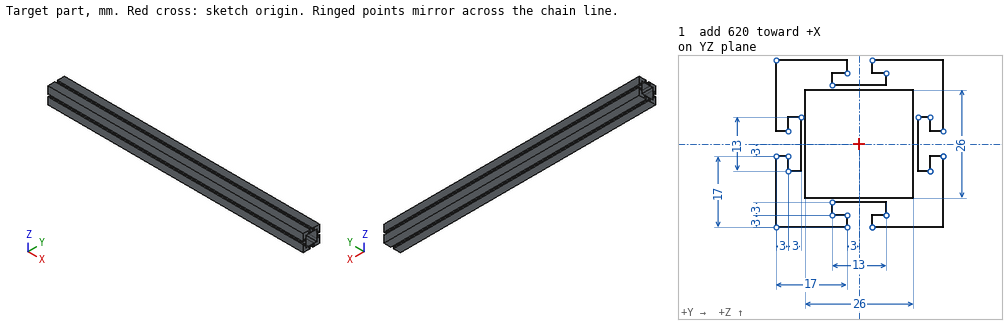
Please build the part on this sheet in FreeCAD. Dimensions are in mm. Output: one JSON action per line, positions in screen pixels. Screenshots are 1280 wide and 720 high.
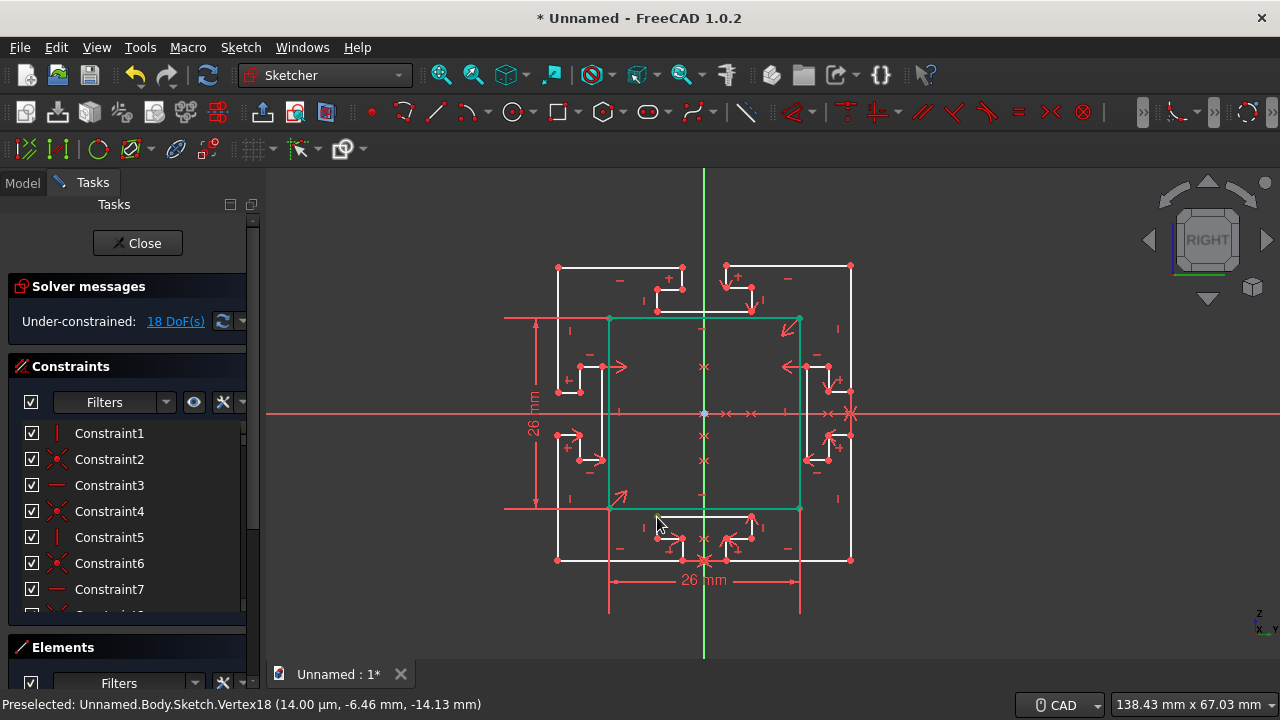
{"action": "left_click", "coordinate": [657, 312]}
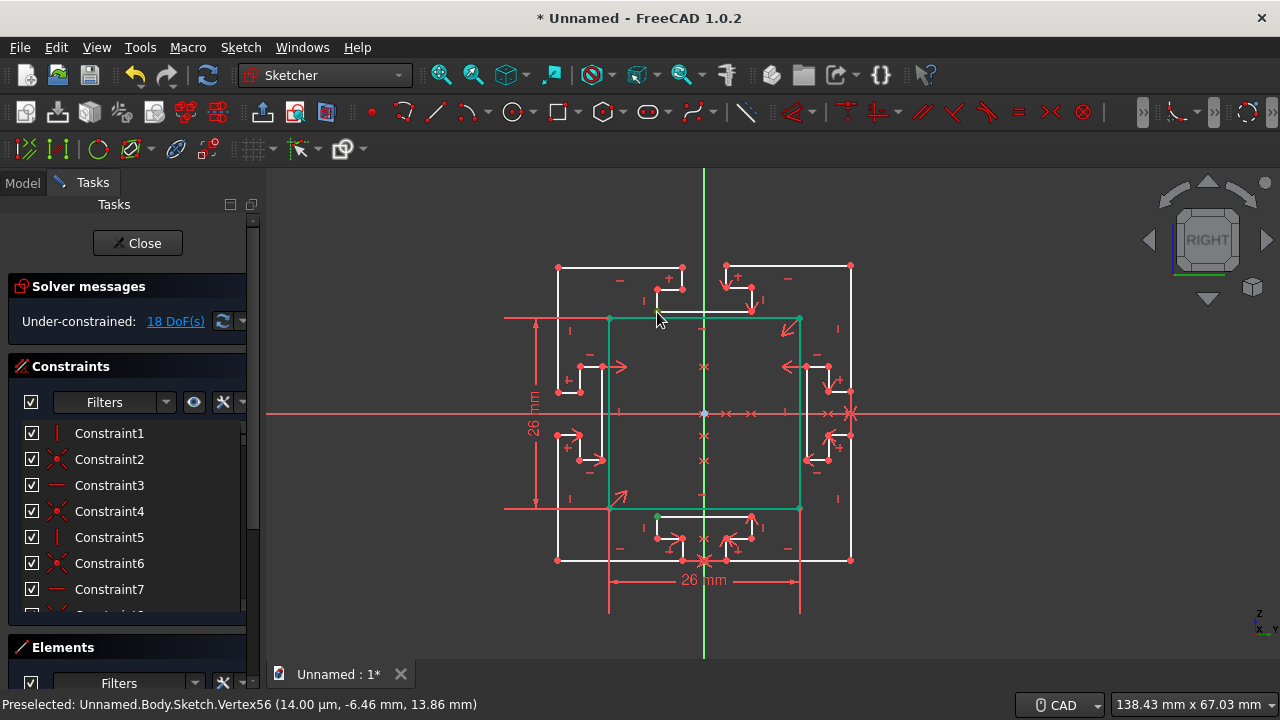
{"action": "left_click", "coordinate": [353, 414]}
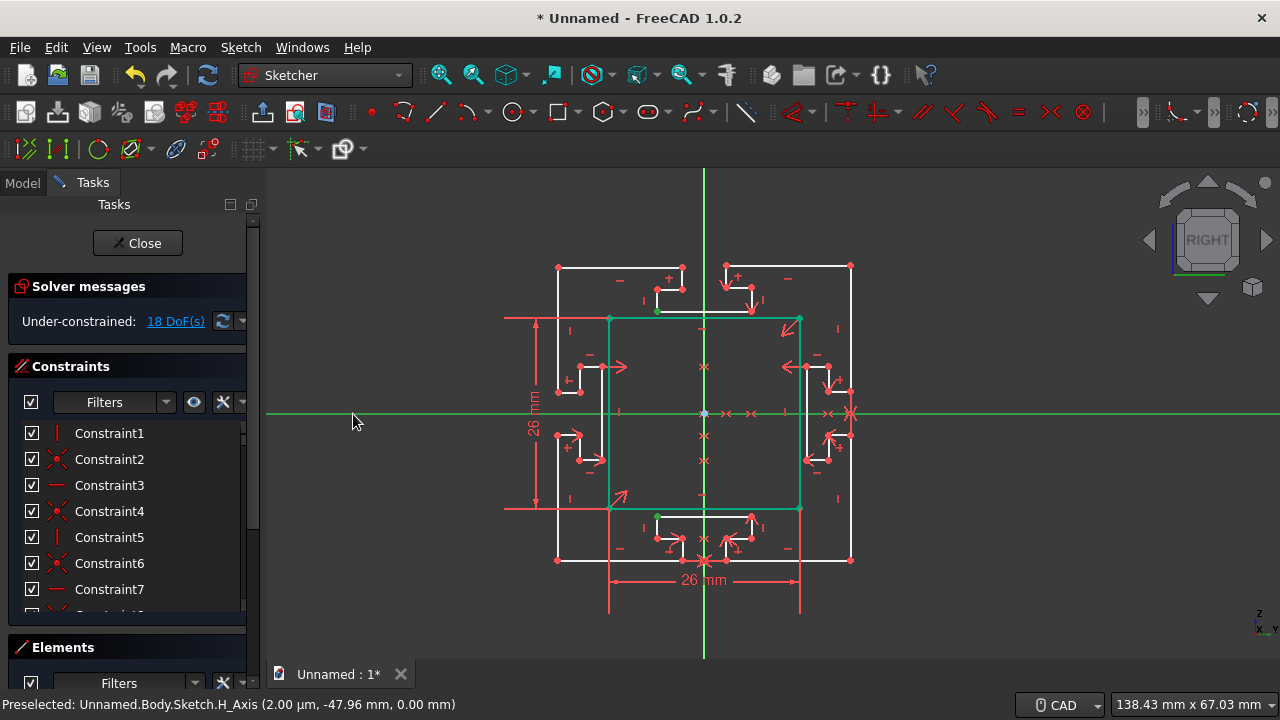
{"action": "left_click", "coordinate": [1052, 112]}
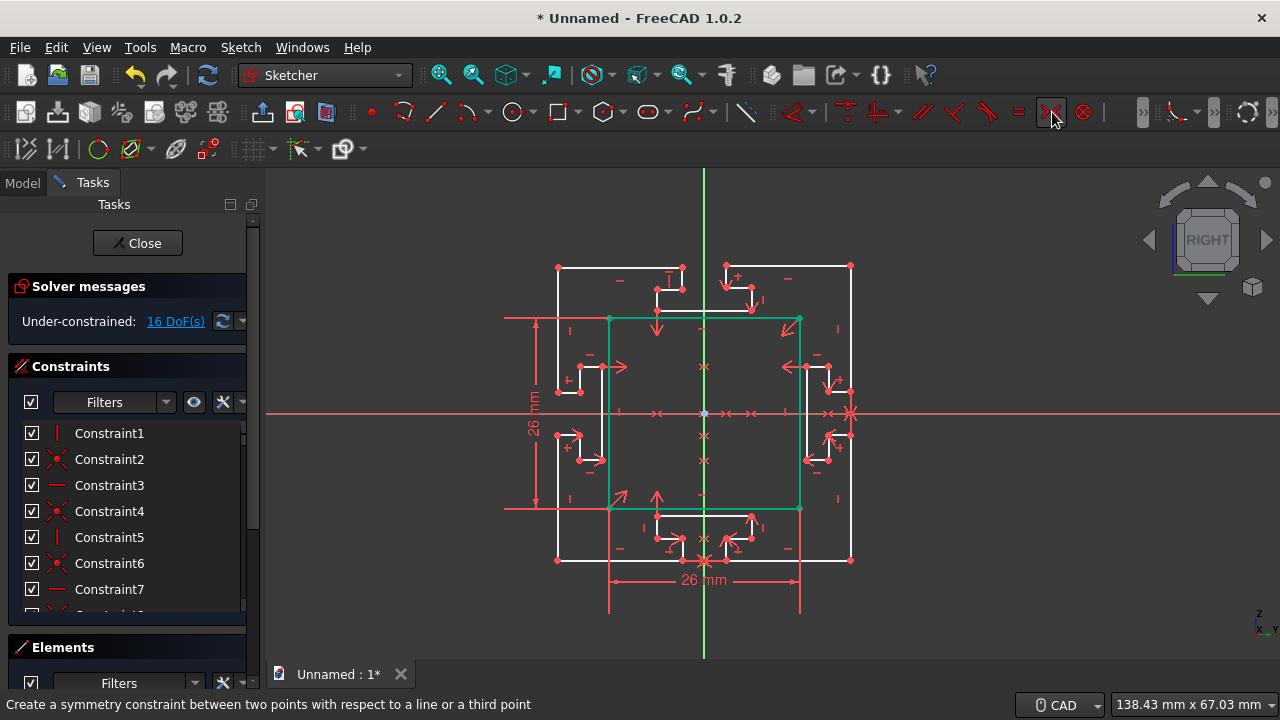
{"action": "left_click", "coordinate": [683, 539]}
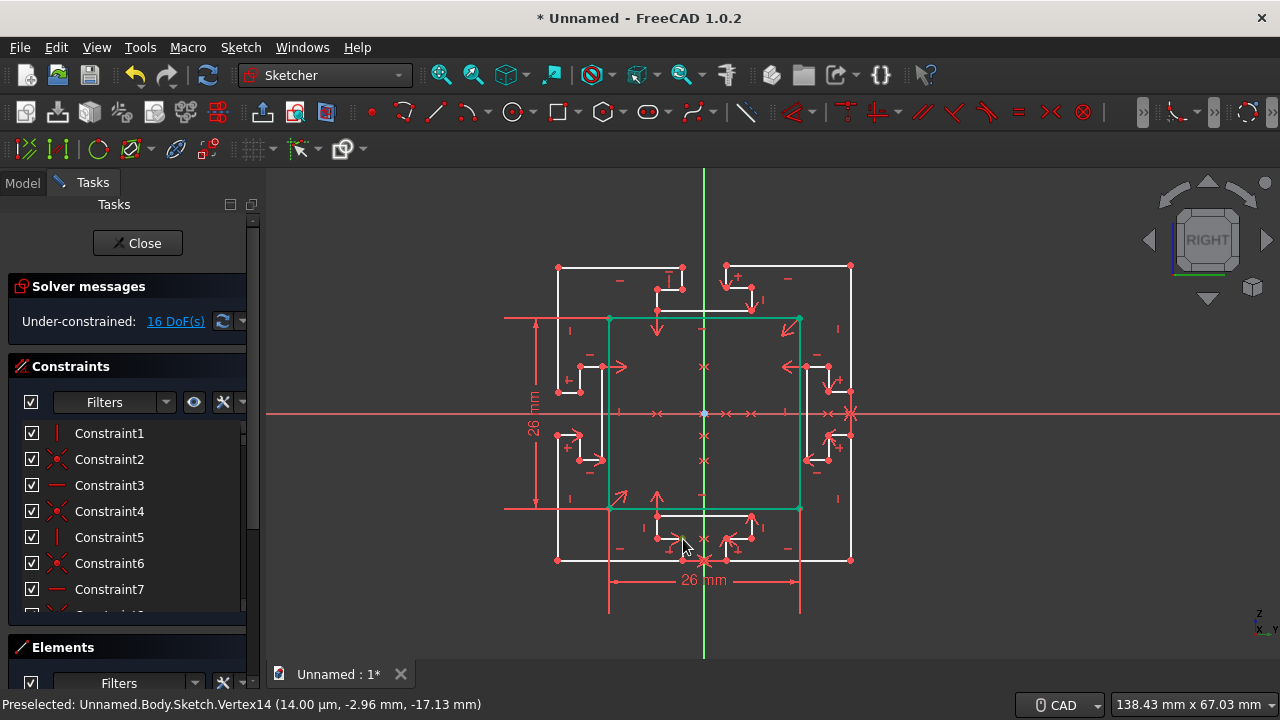
{"action": "left_click", "coordinate": [682, 290]}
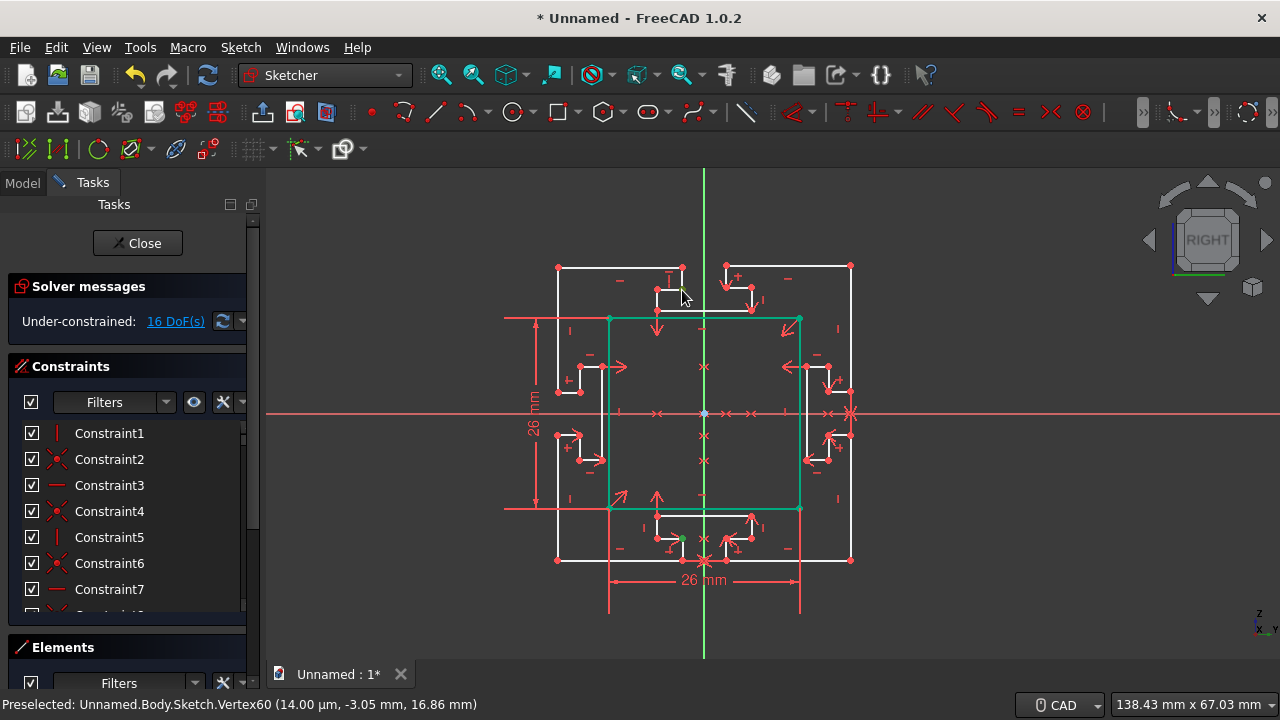
{"action": "left_click", "coordinate": [353, 414]}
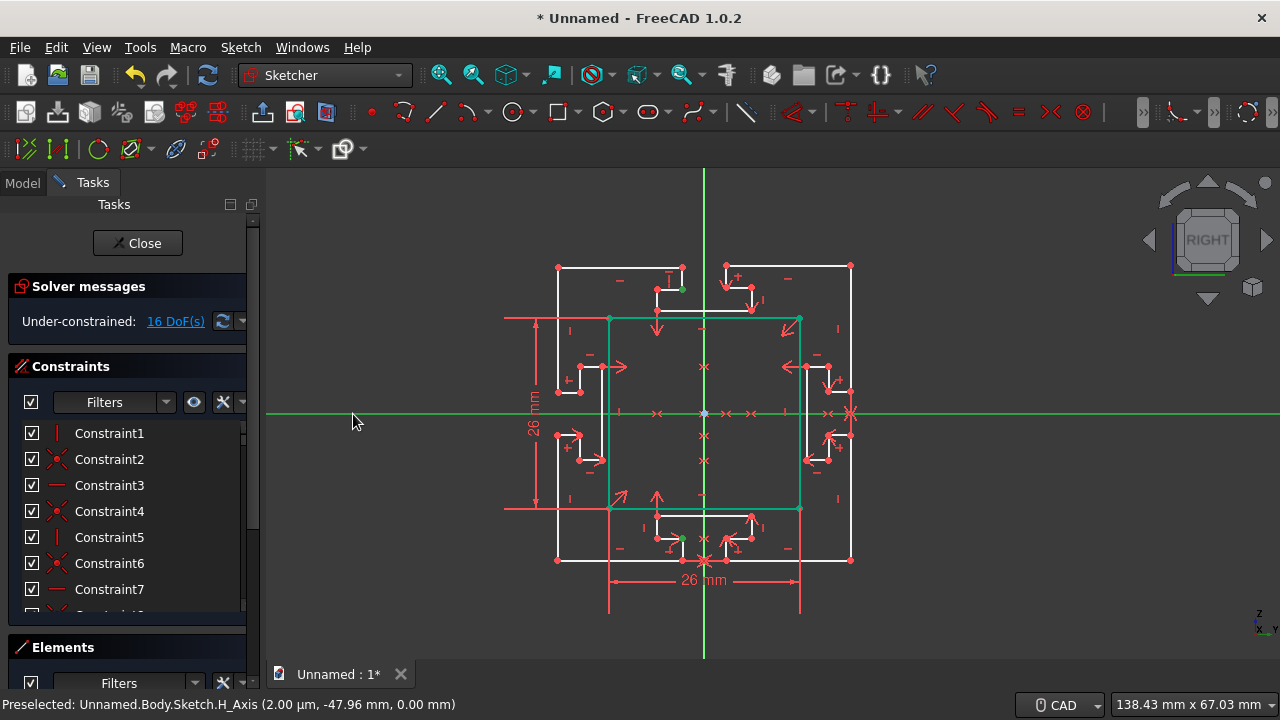
{"action": "key", "text": "s"}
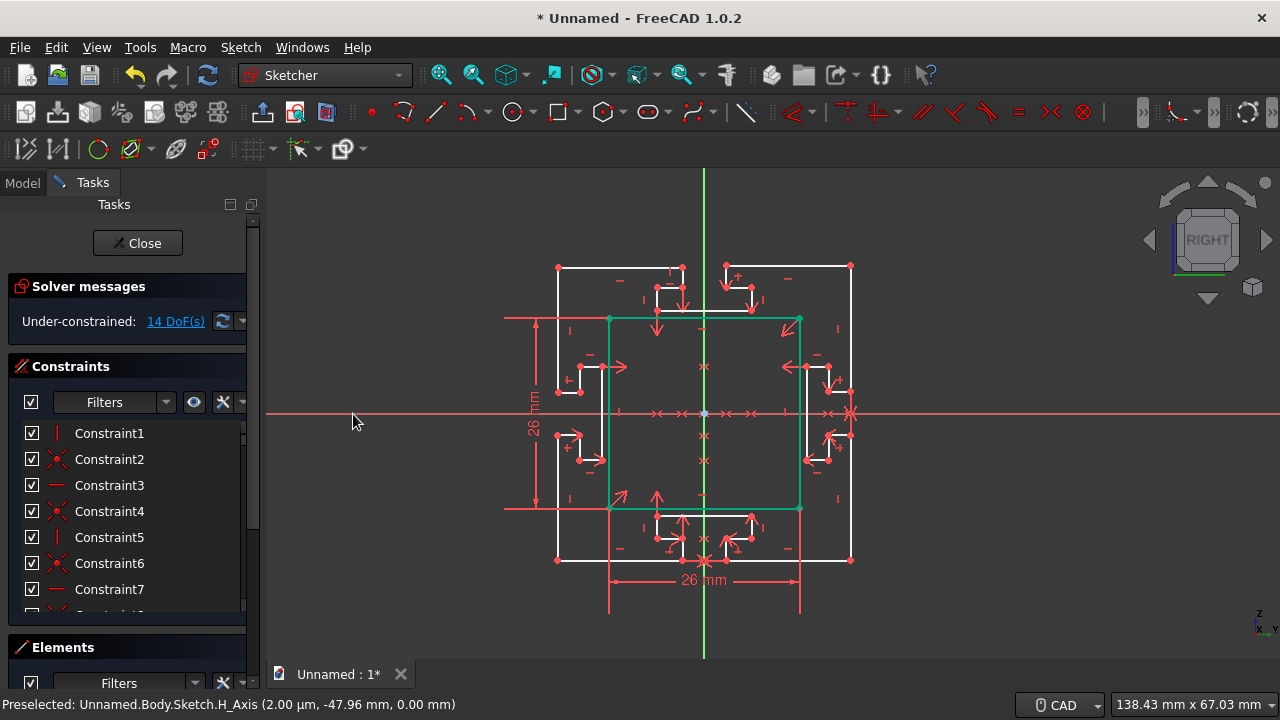
{"action": "left_click", "coordinate": [558, 561]}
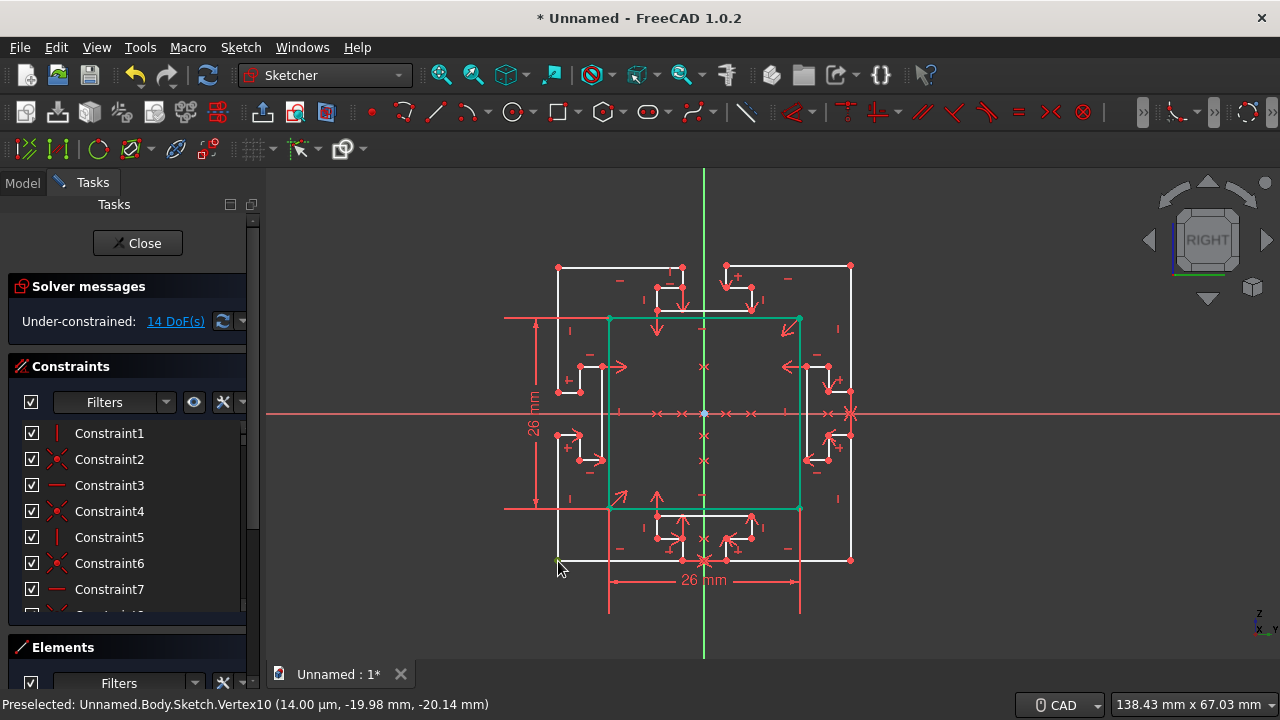
{"action": "left_click", "coordinate": [558, 268]}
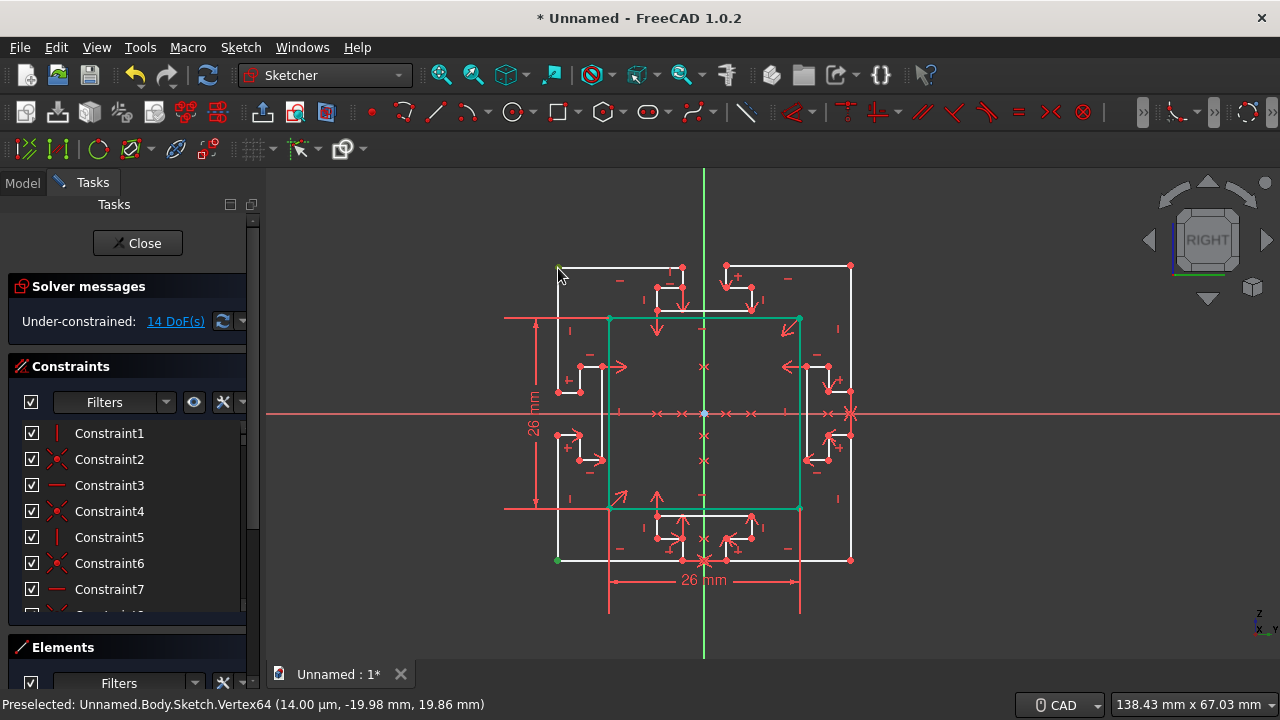
{"action": "left_click", "coordinate": [353, 414]}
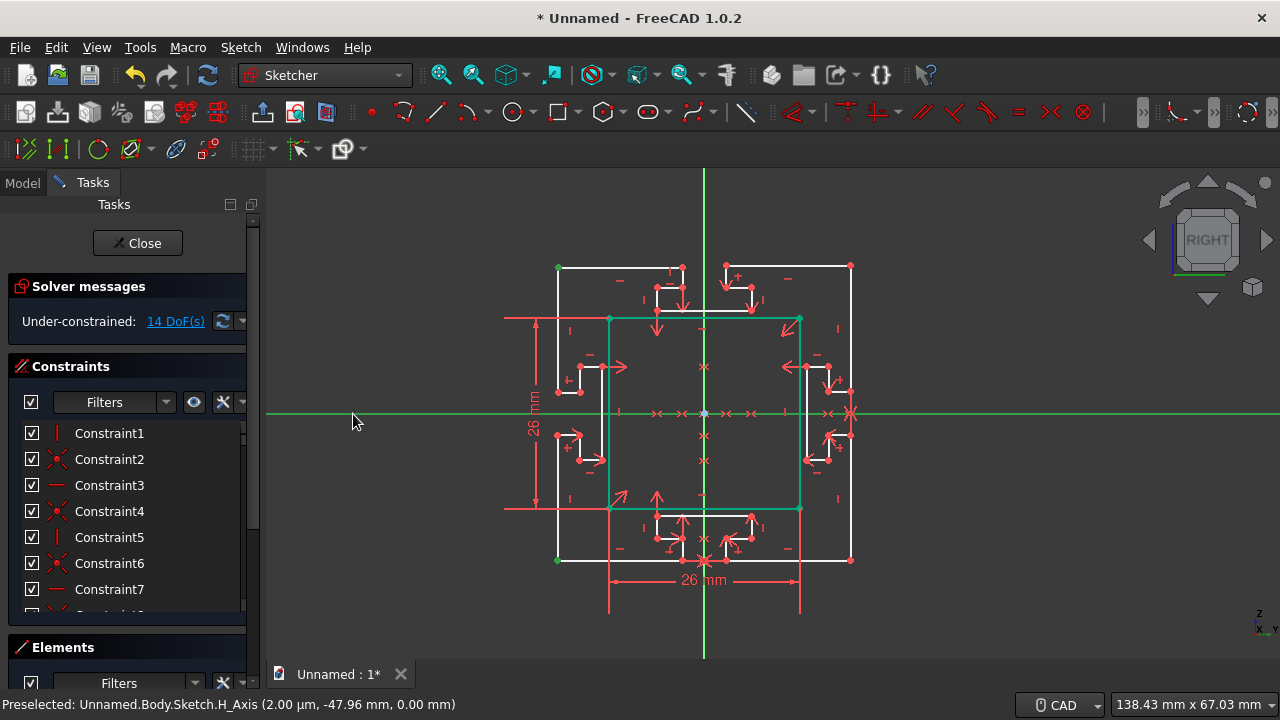
{"action": "left_click", "coordinate": [1052, 112]}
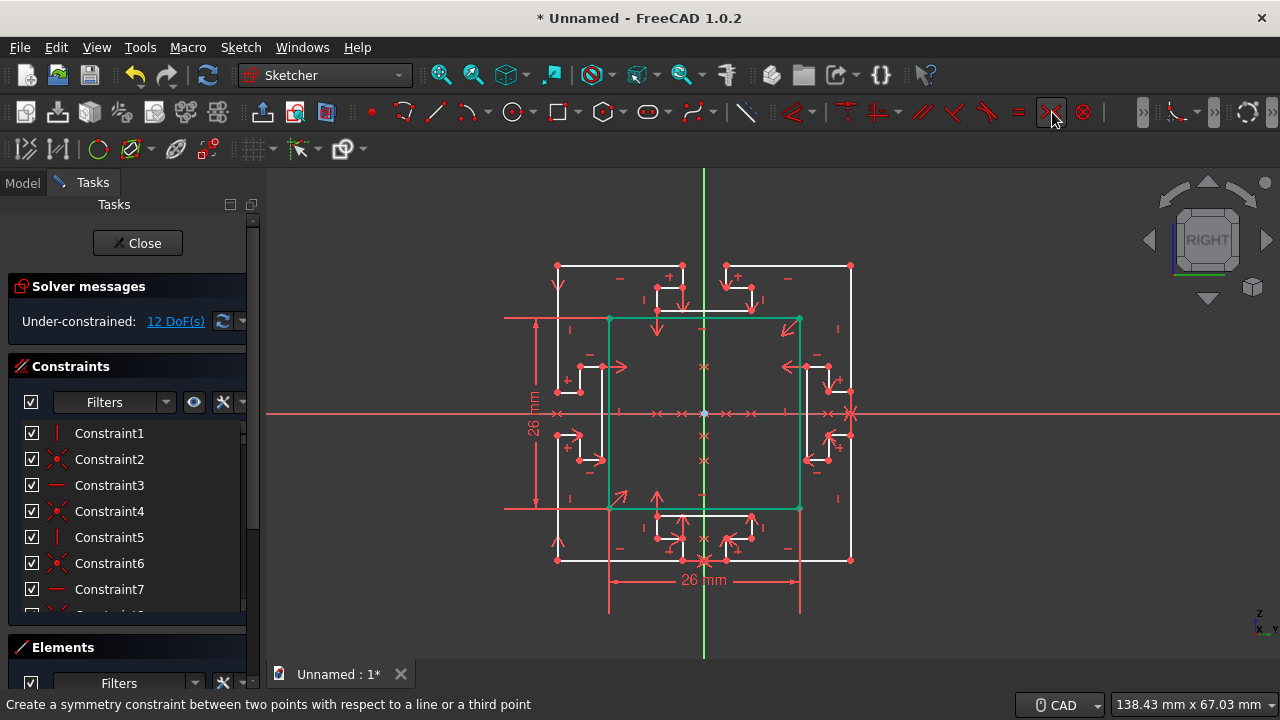
{"action": "left_click", "coordinate": [580, 435]}